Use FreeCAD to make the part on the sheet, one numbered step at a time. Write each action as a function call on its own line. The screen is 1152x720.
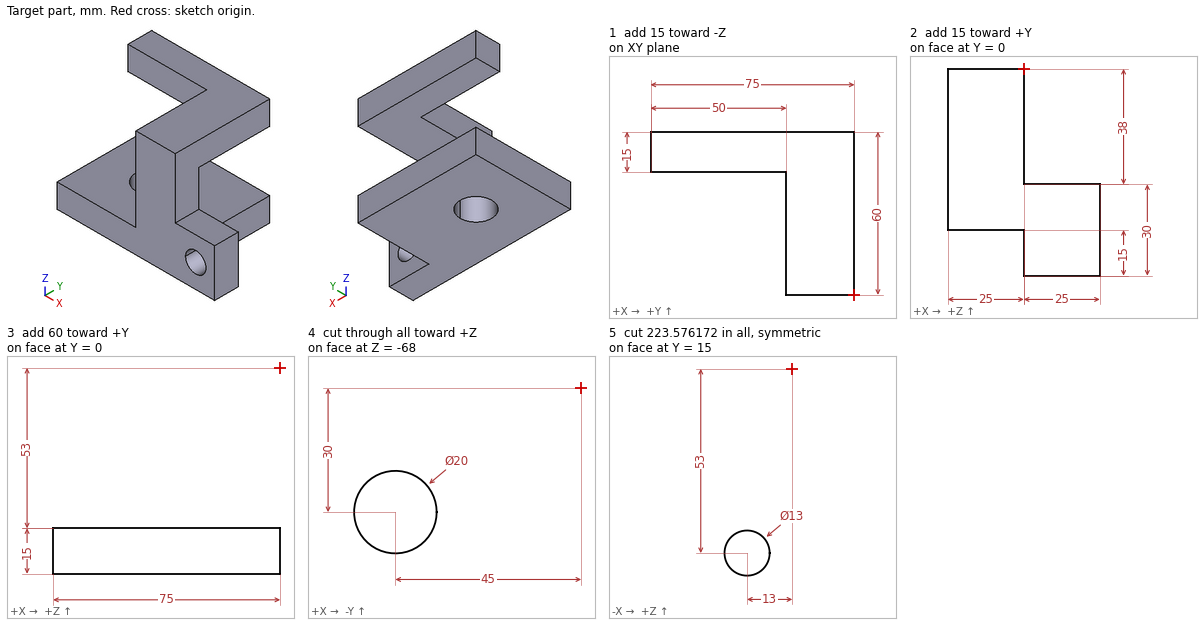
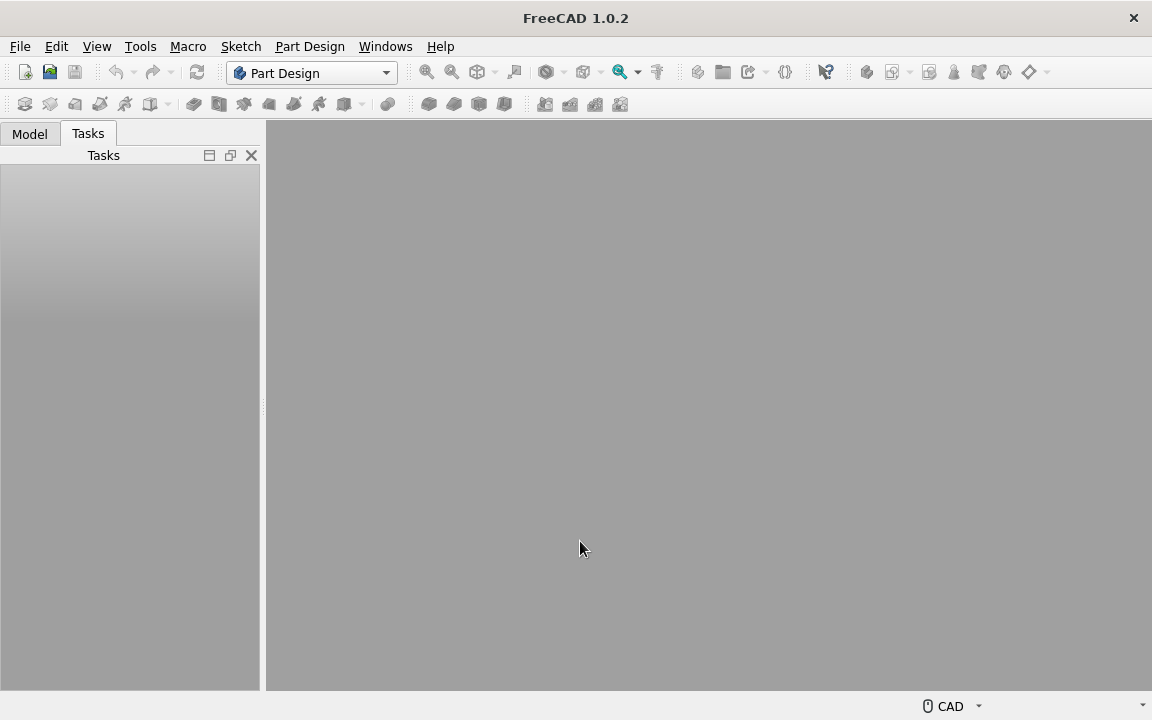
click(25, 72)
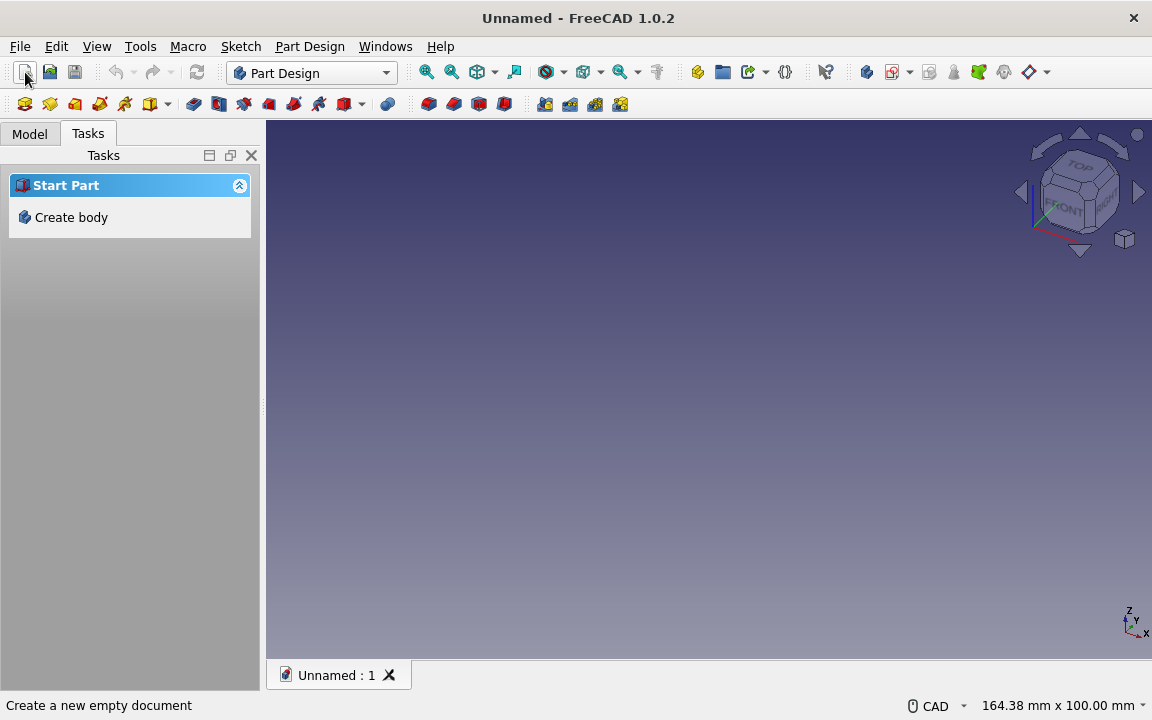
click(892, 72)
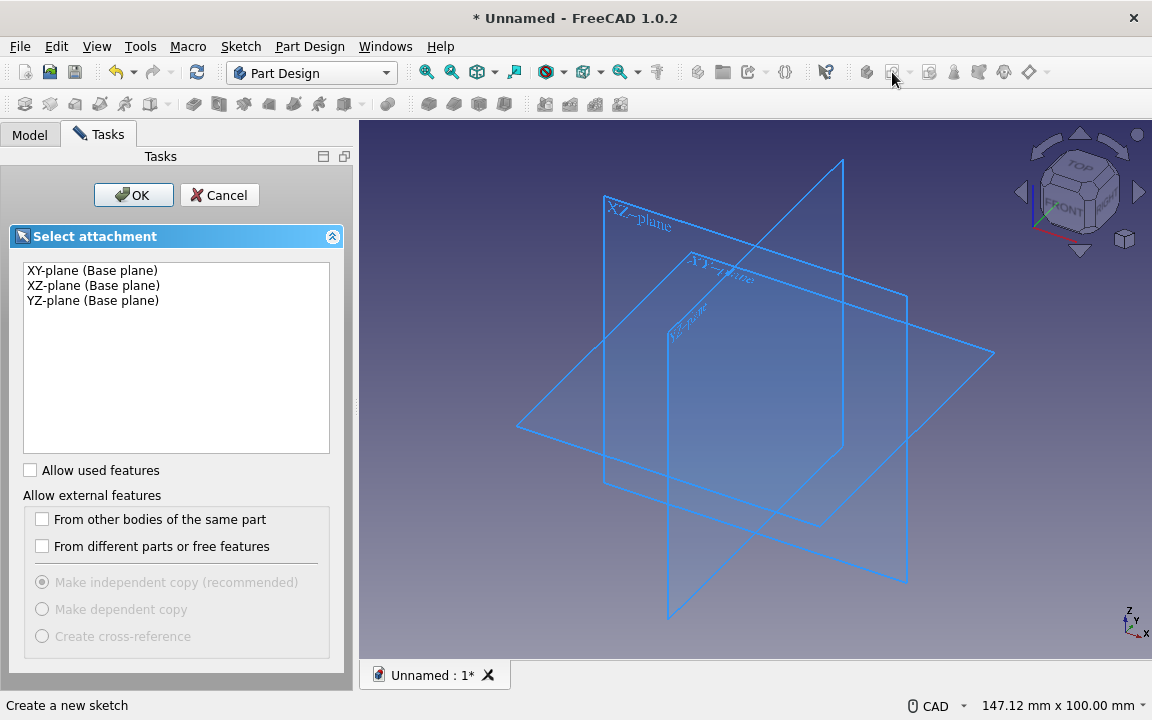
click(84, 270)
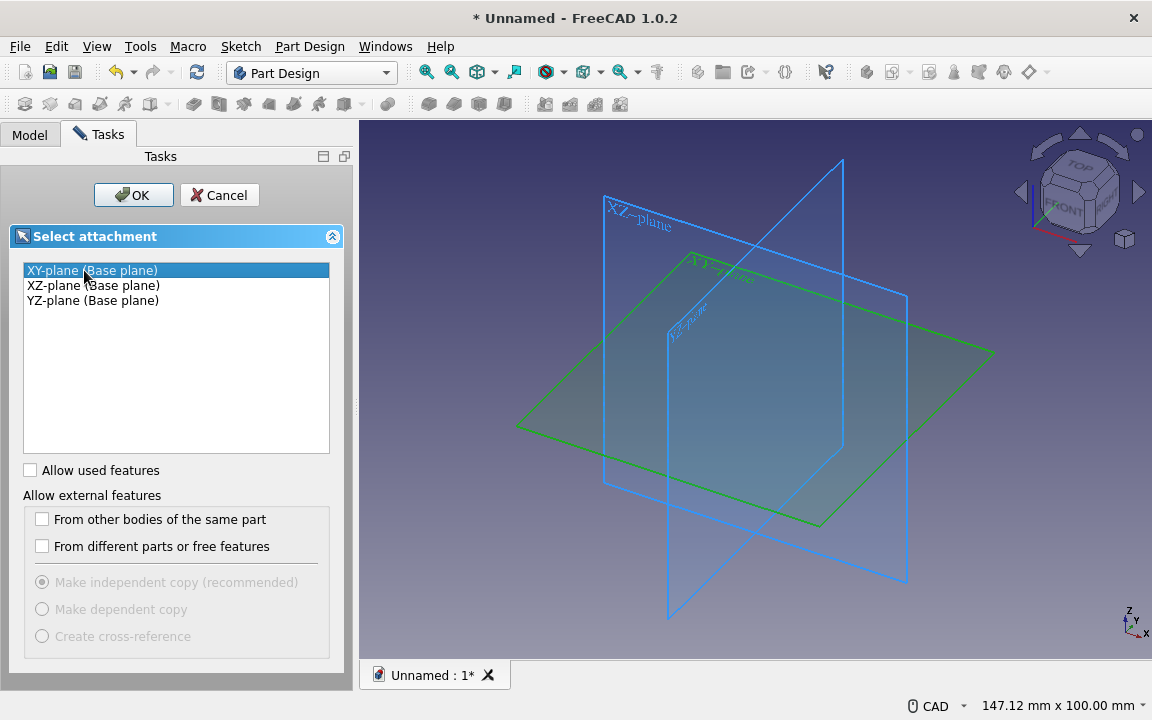
click(134, 195)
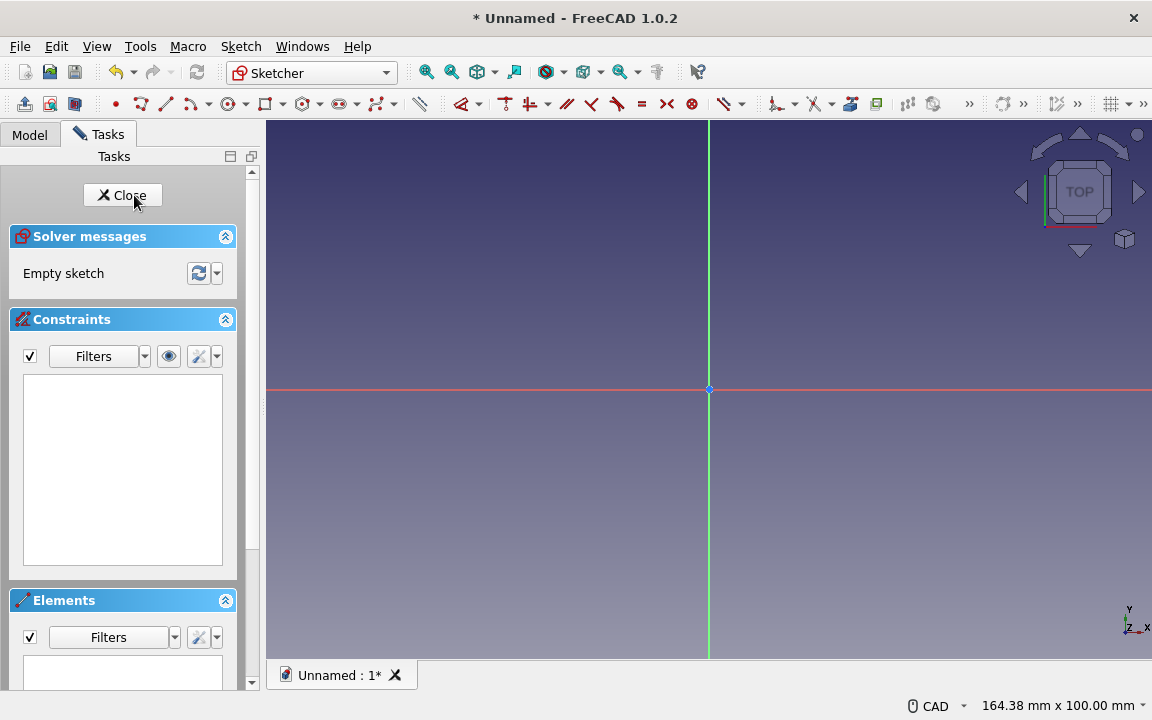
scroll(912, 631, down, 2)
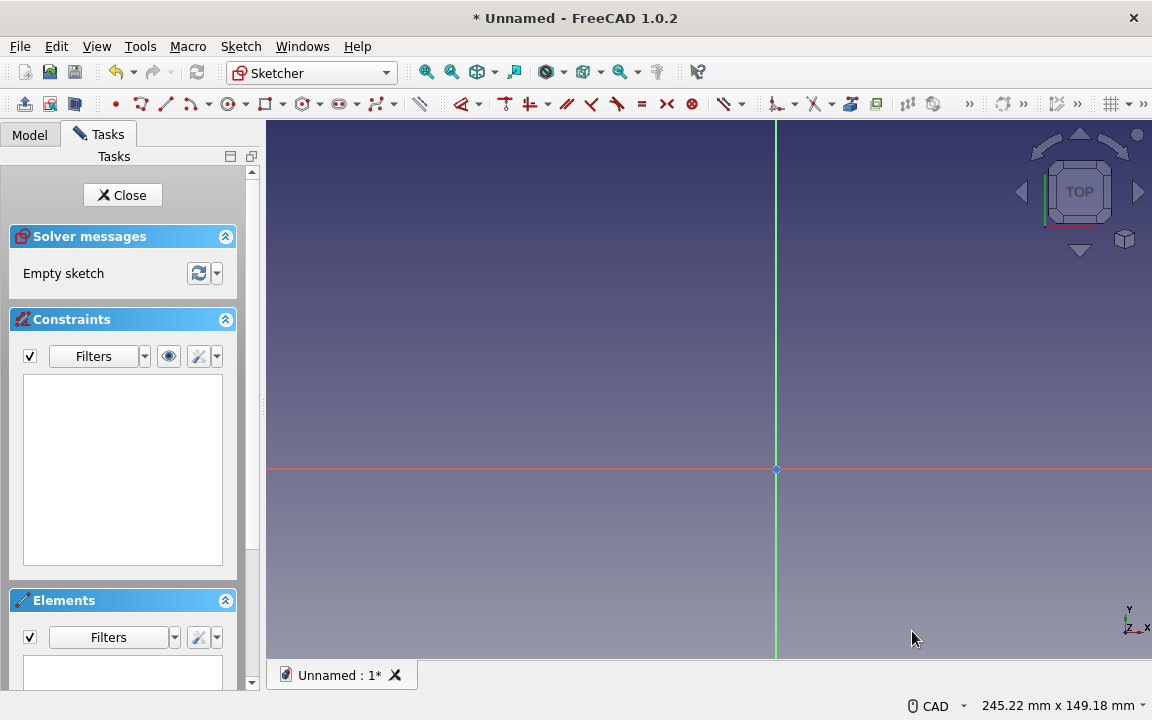
scroll(641, 303, up, 2)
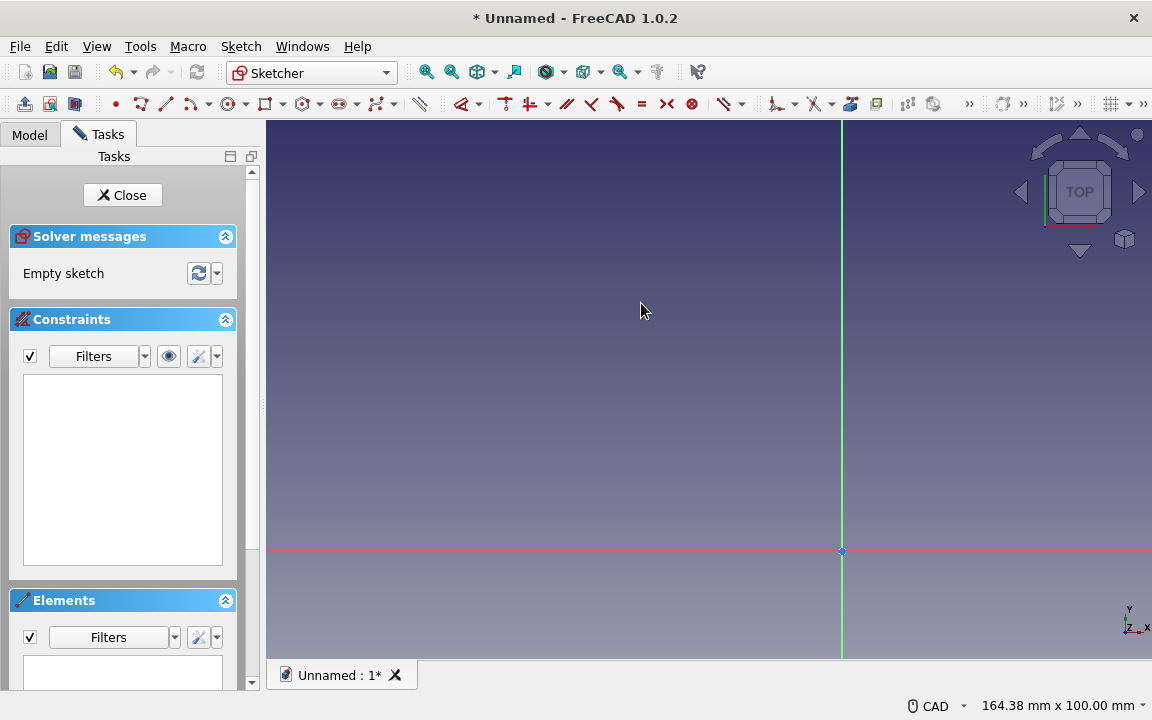
click(141, 104)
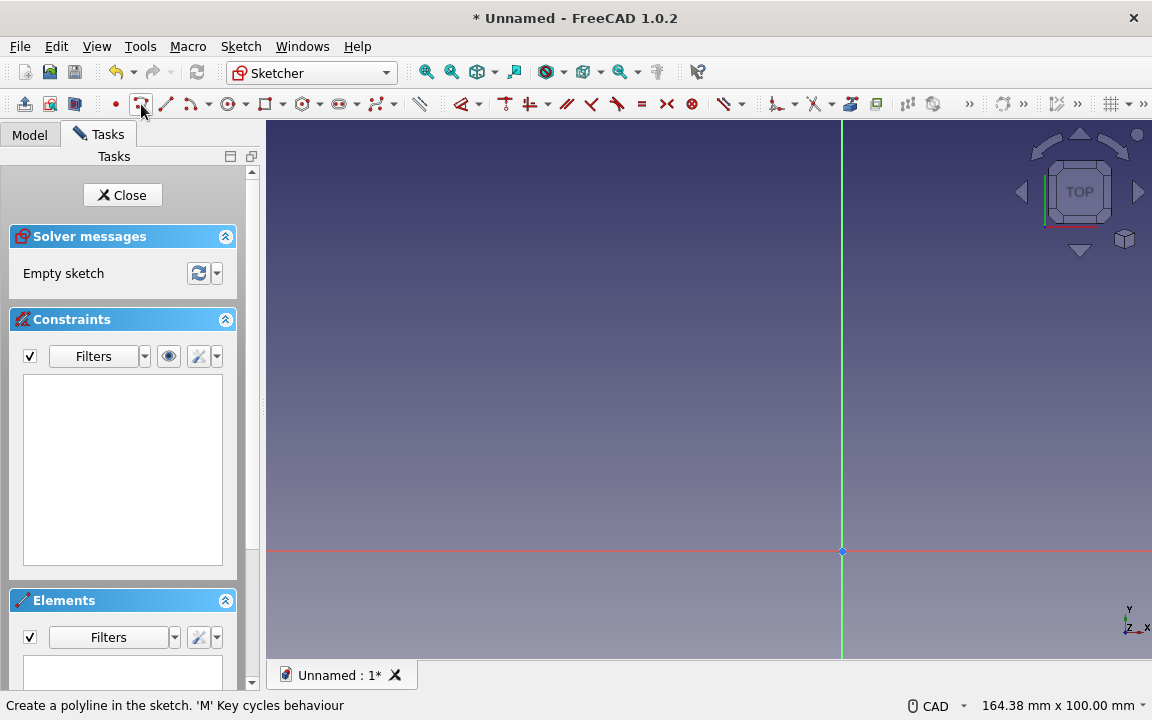
click(842, 551)
click(833, 228)
click(438, 228)
click(438, 309)
click(708, 309)
click(708, 542)
click(842, 551)
key(Escape)
key(Escape)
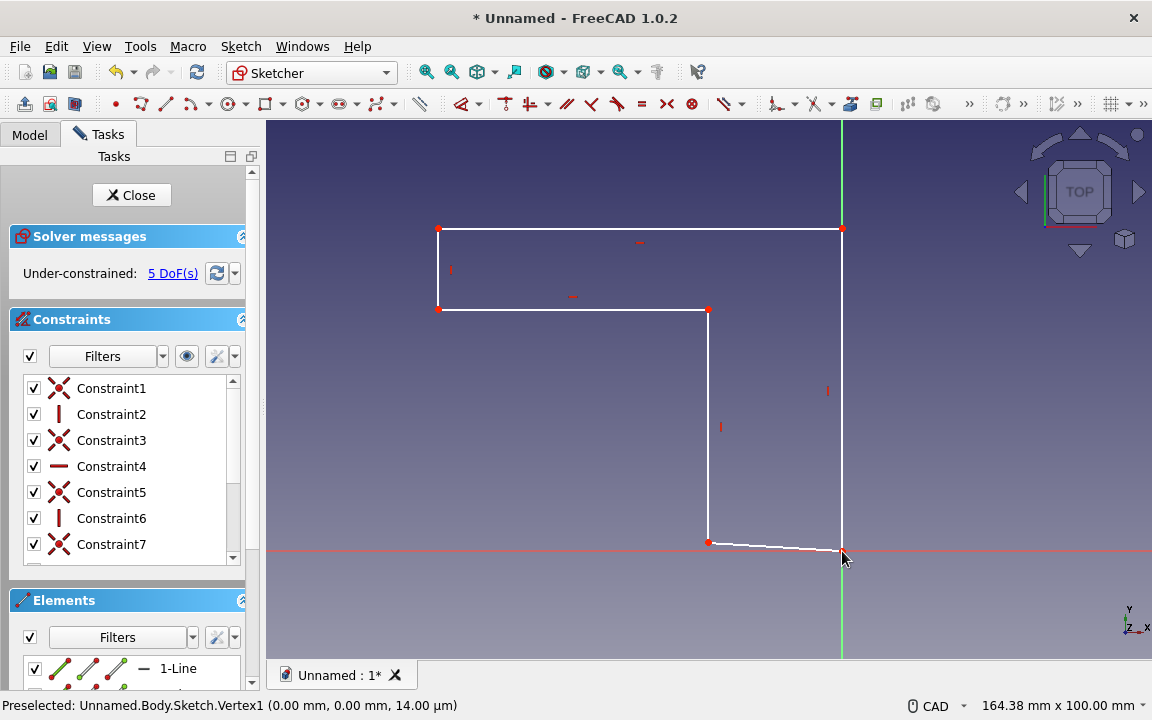
click(802, 549)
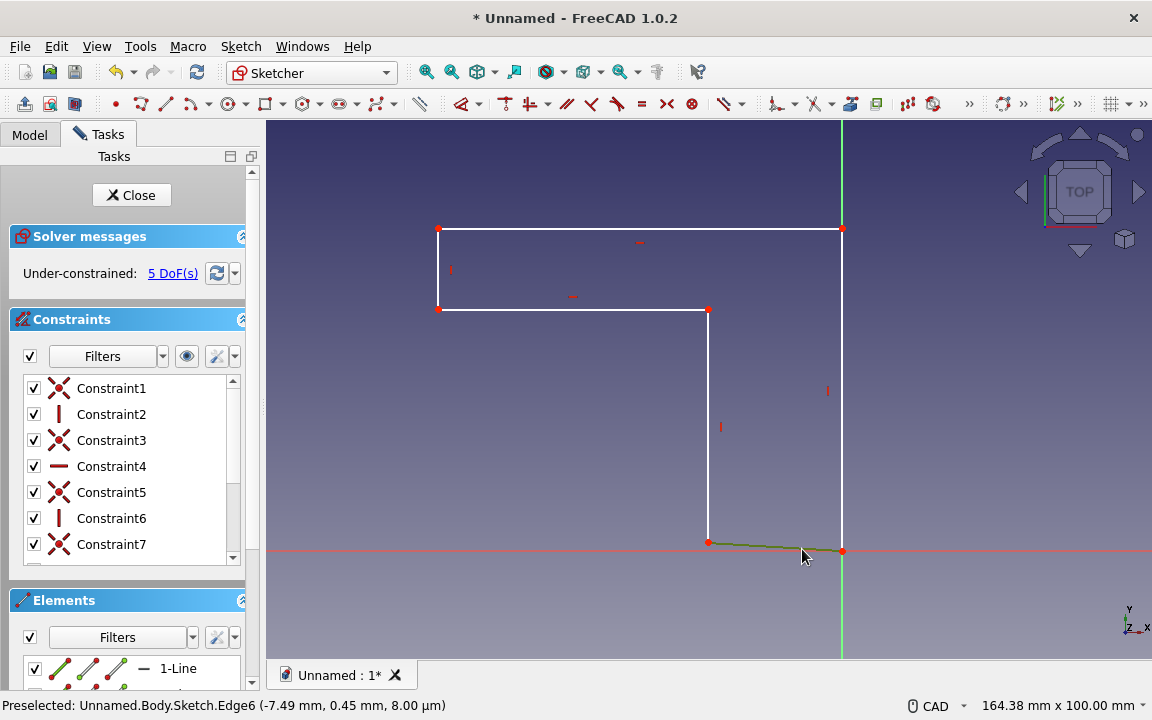
key(h)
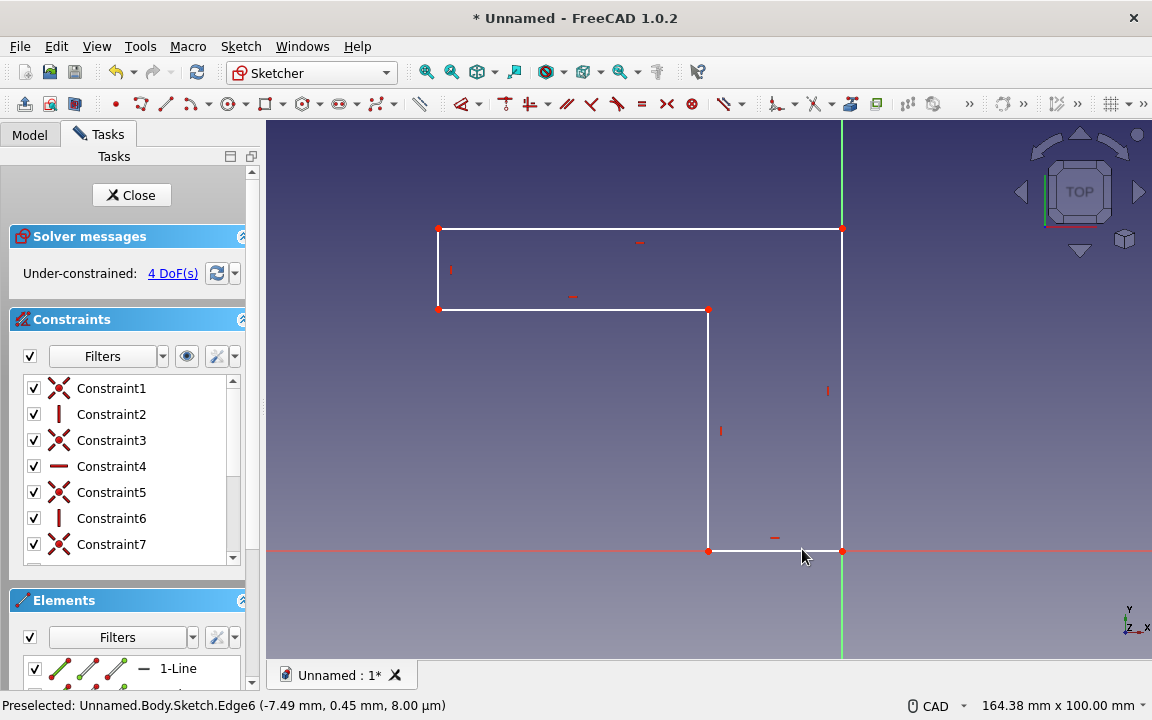
click(460, 104)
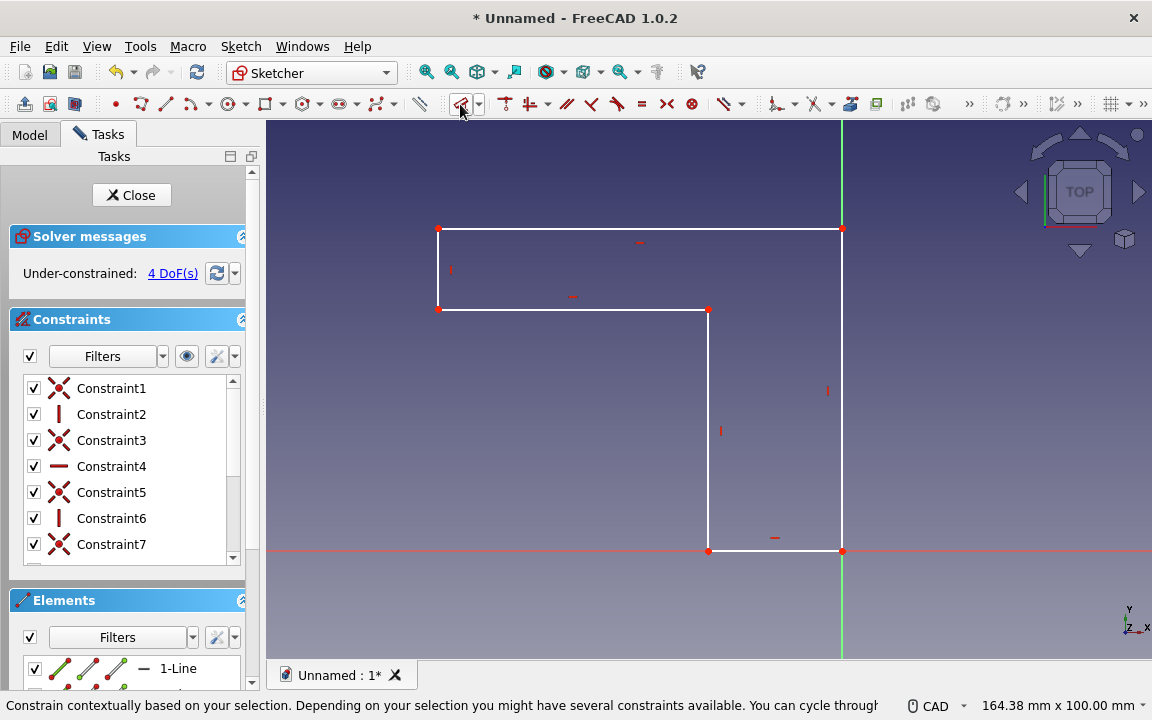
click(842, 454)
click(876, 390)